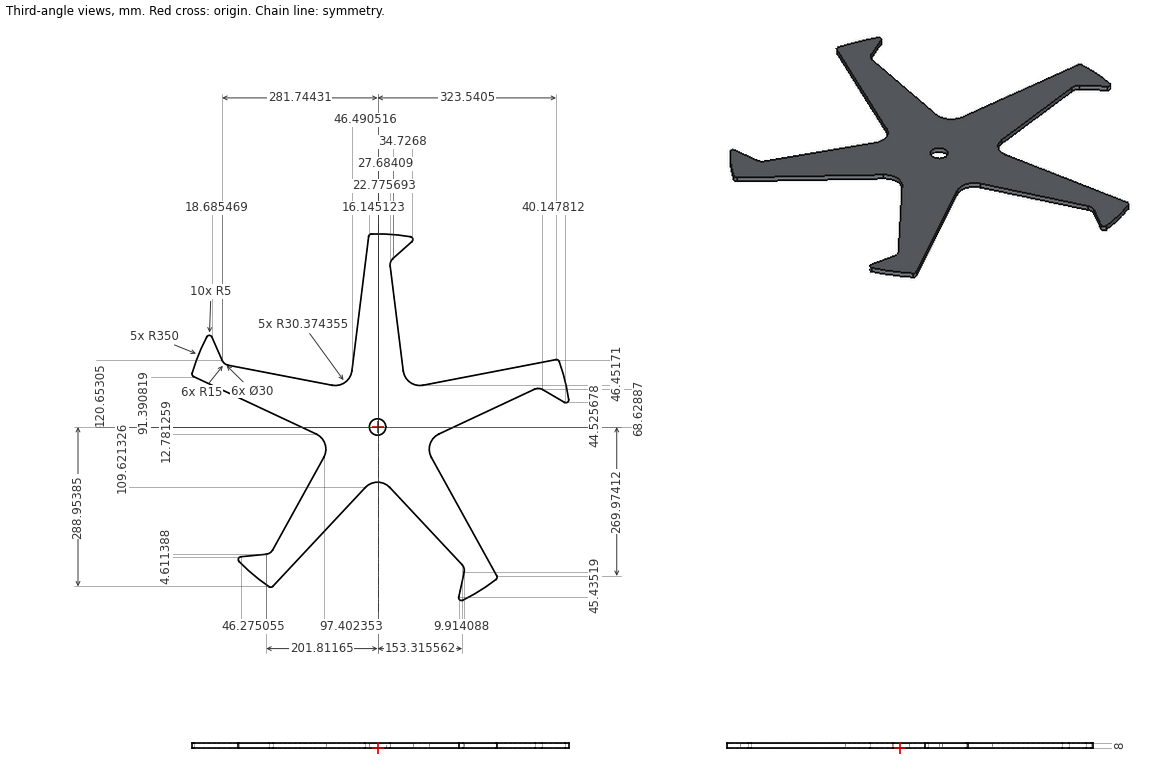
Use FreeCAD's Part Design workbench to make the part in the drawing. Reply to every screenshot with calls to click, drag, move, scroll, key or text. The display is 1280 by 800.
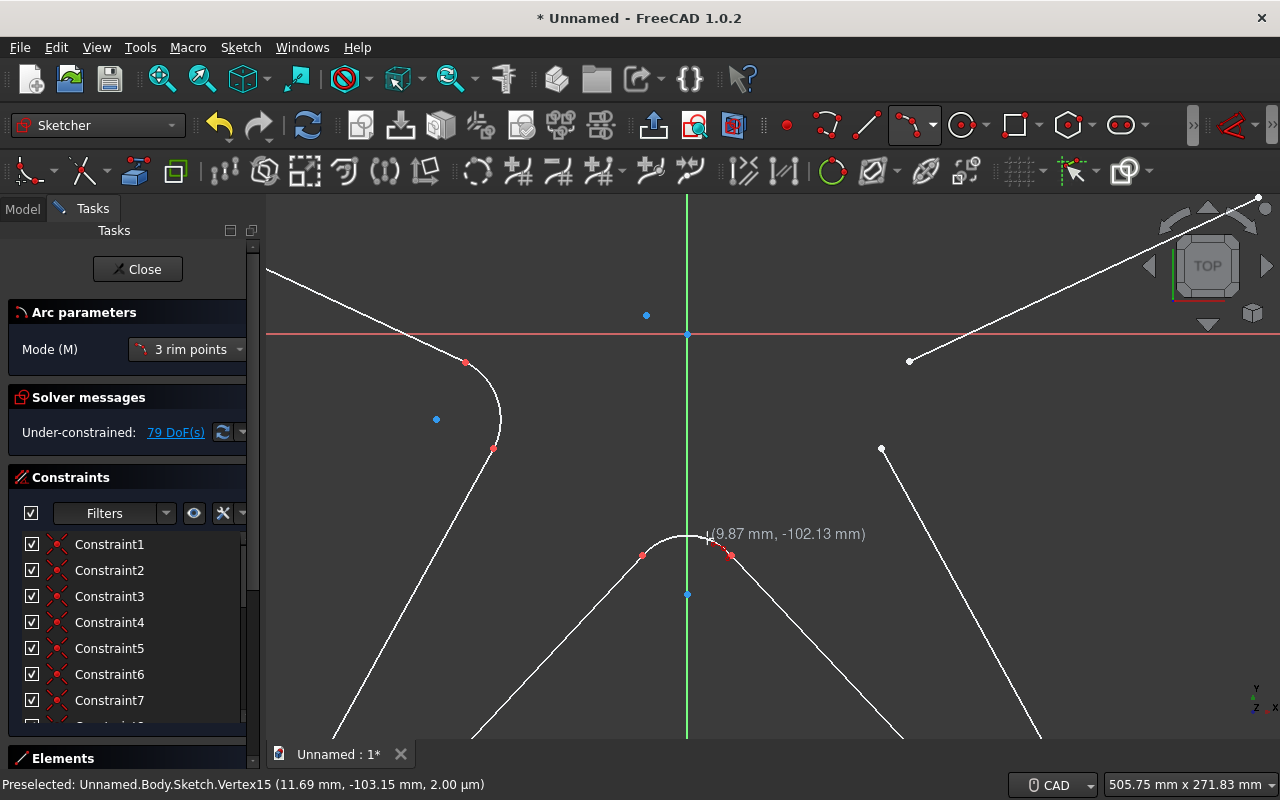
scroll(707, 521, down, 7)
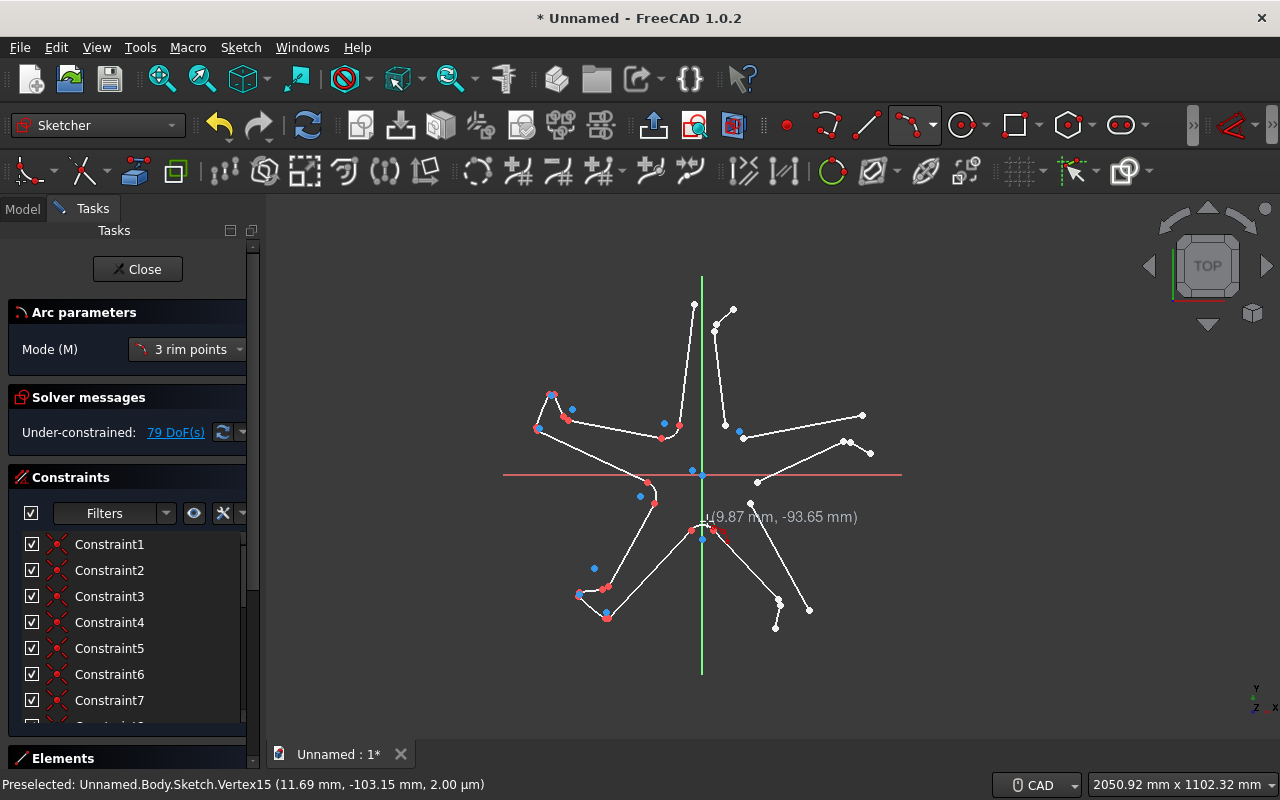
scroll(778, 599, up, 5)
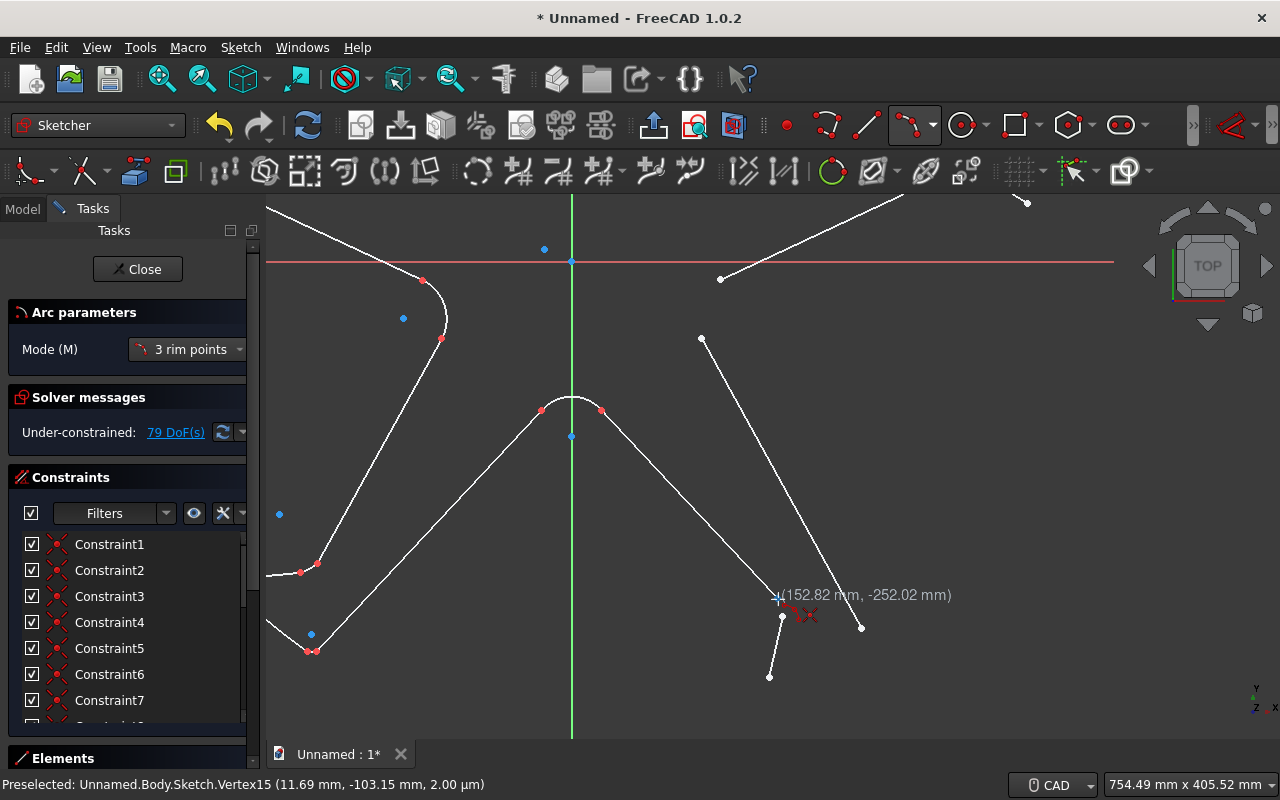
click(778, 599)
click(783, 617)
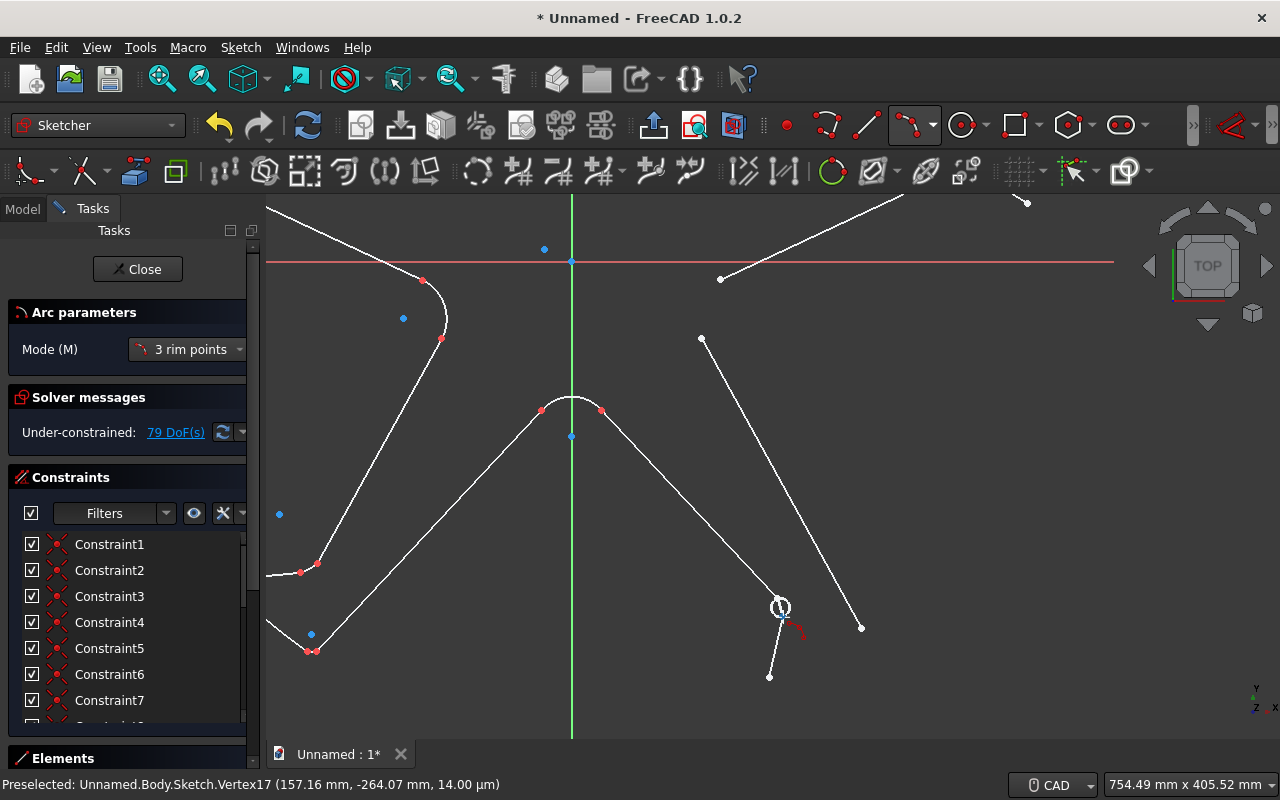
scroll(783, 606, up, 10)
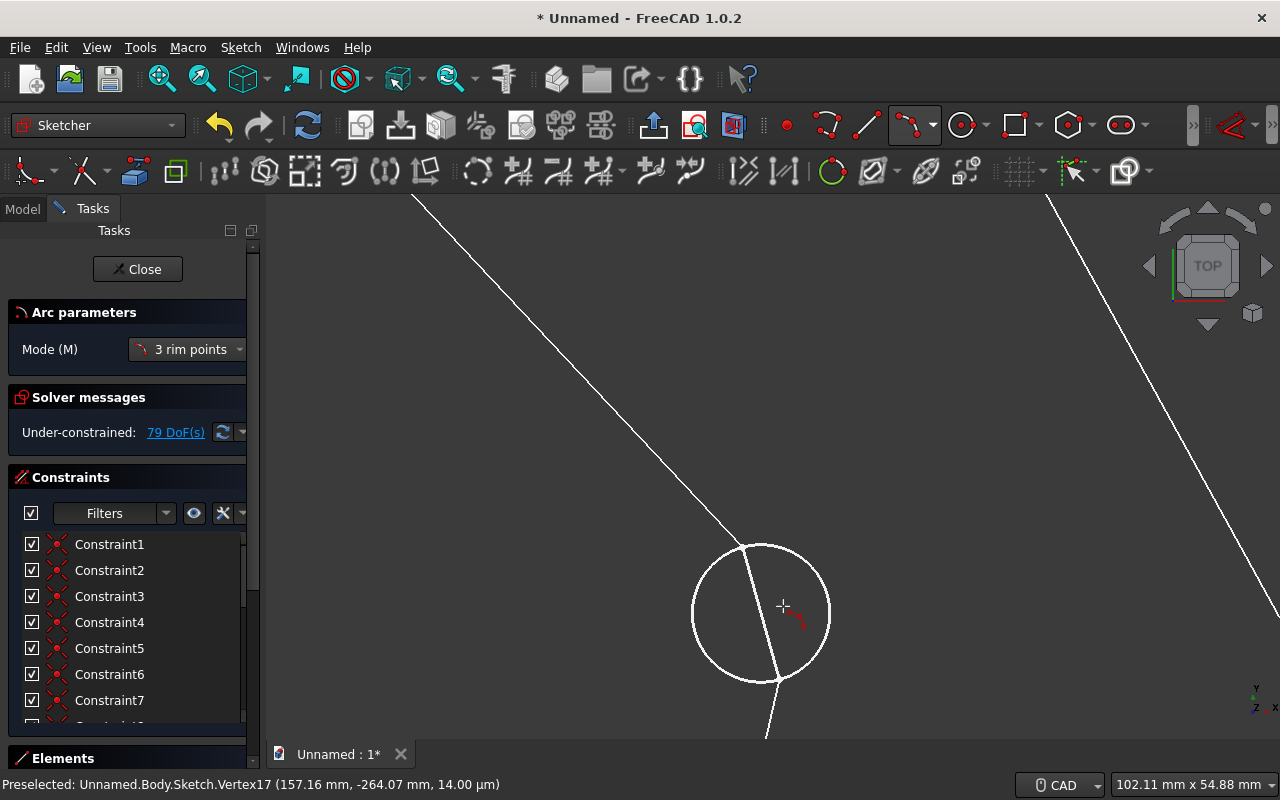
click(776, 600)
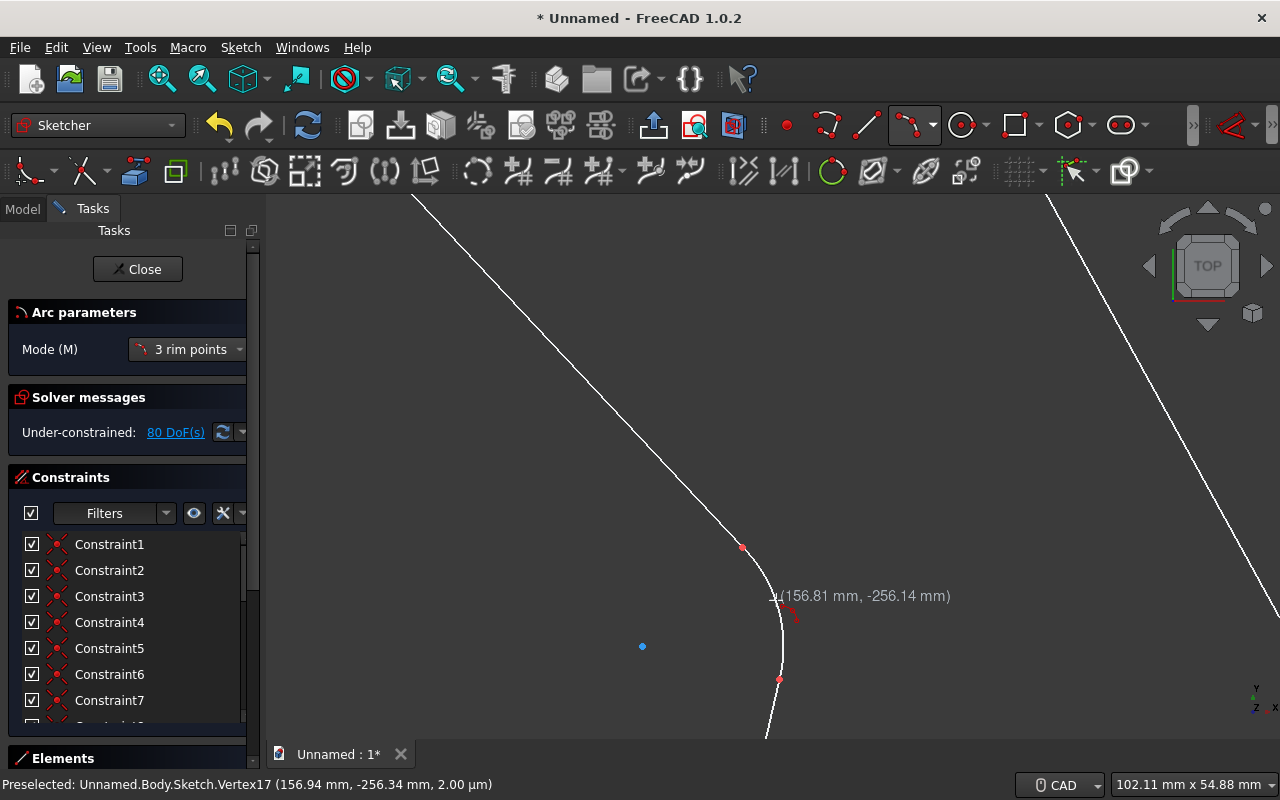
scroll(780, 602, down, 15)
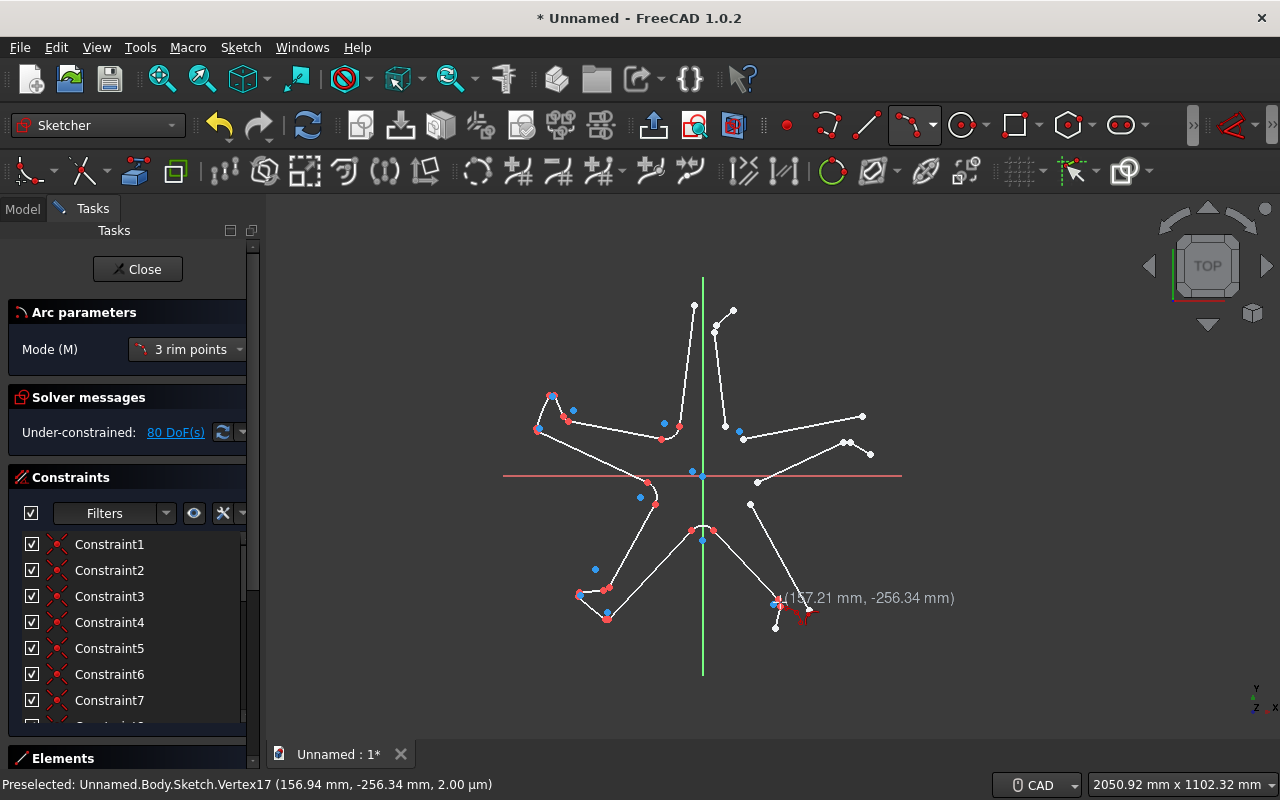
scroll(775, 629, up, 2)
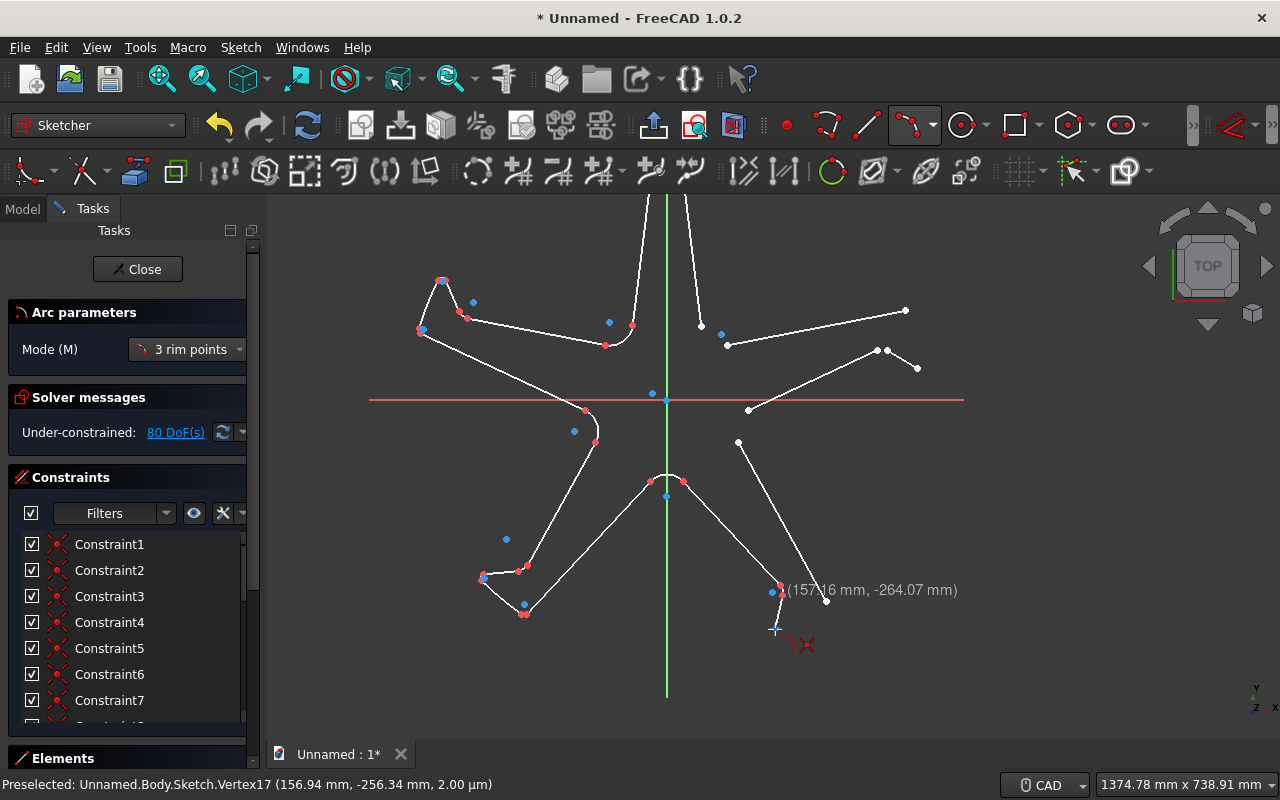
click(775, 629)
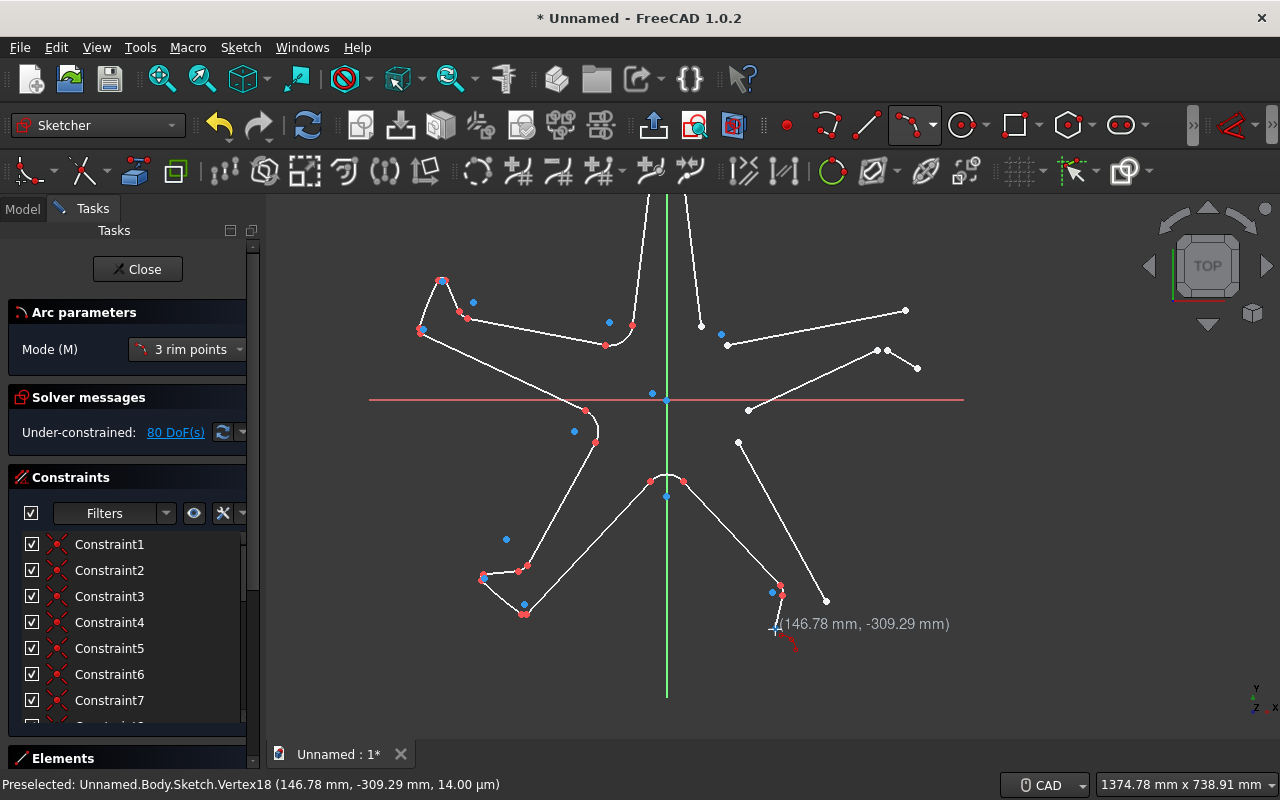
scroll(781, 632, up, 5)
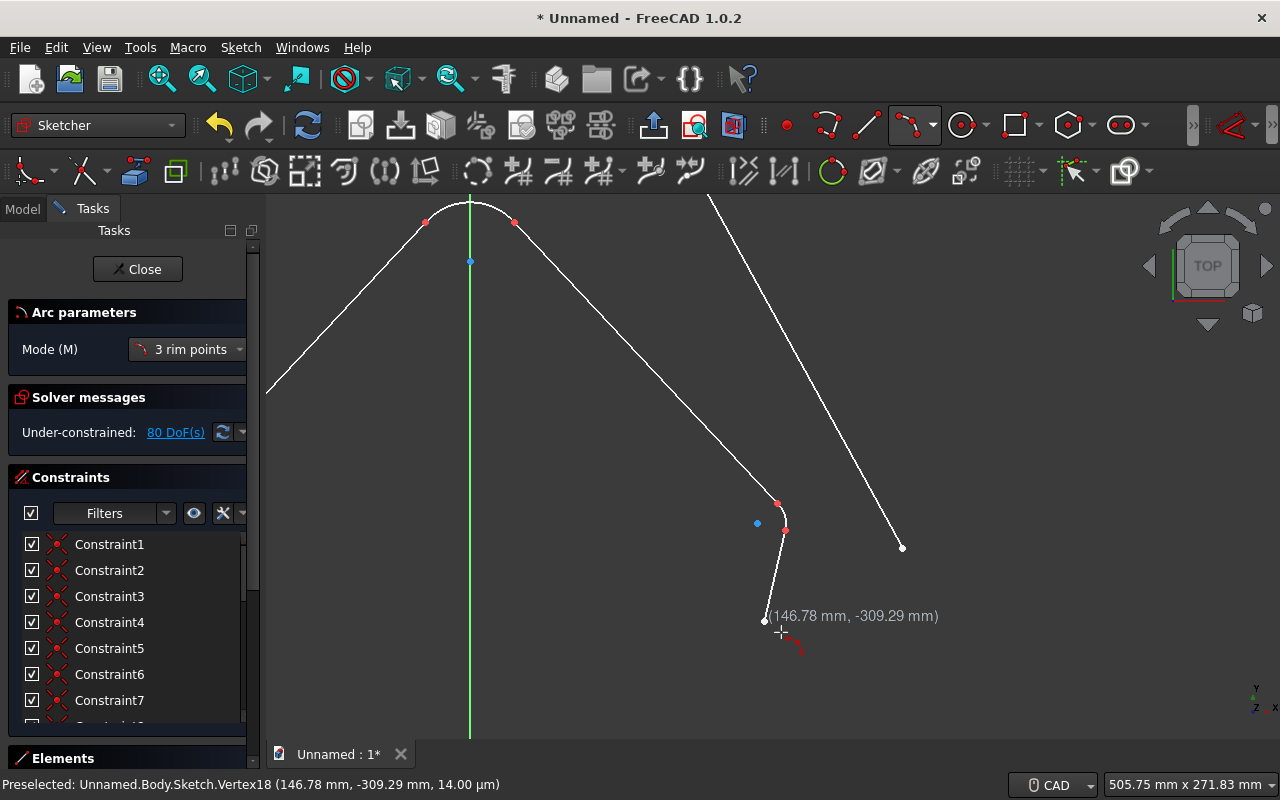
click(779, 631)